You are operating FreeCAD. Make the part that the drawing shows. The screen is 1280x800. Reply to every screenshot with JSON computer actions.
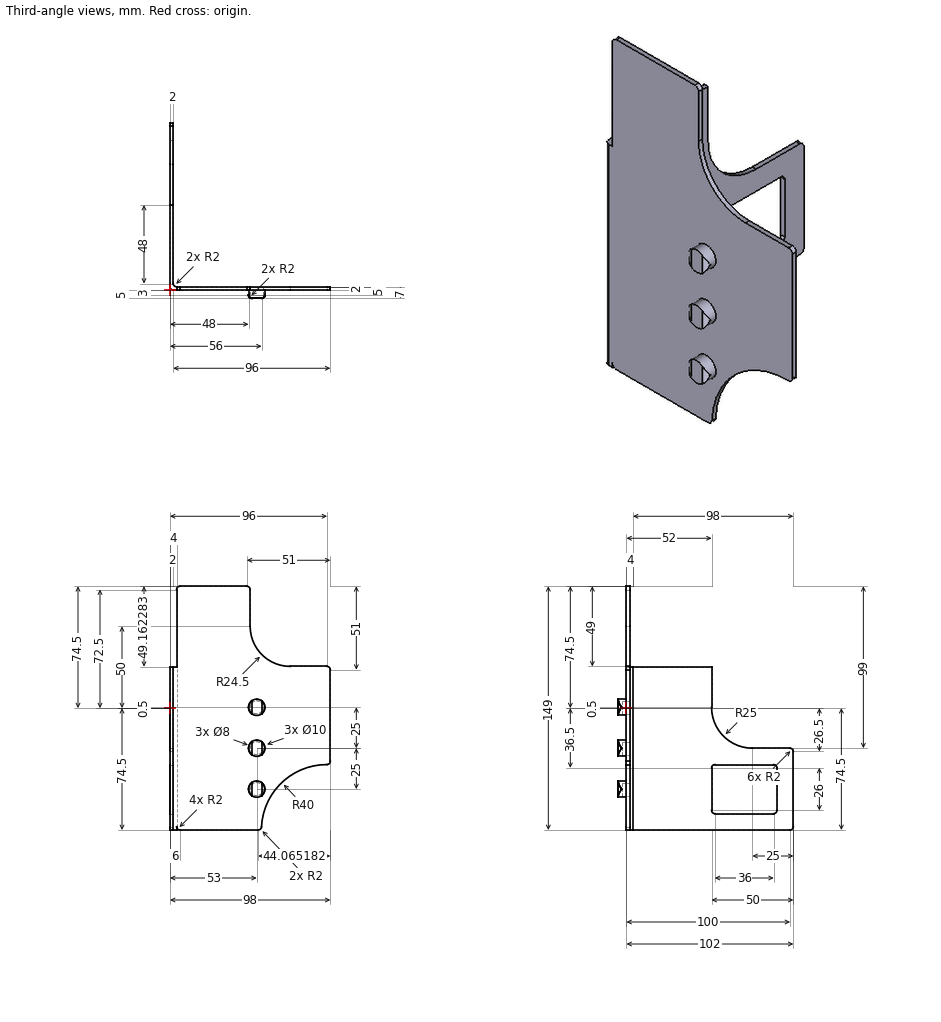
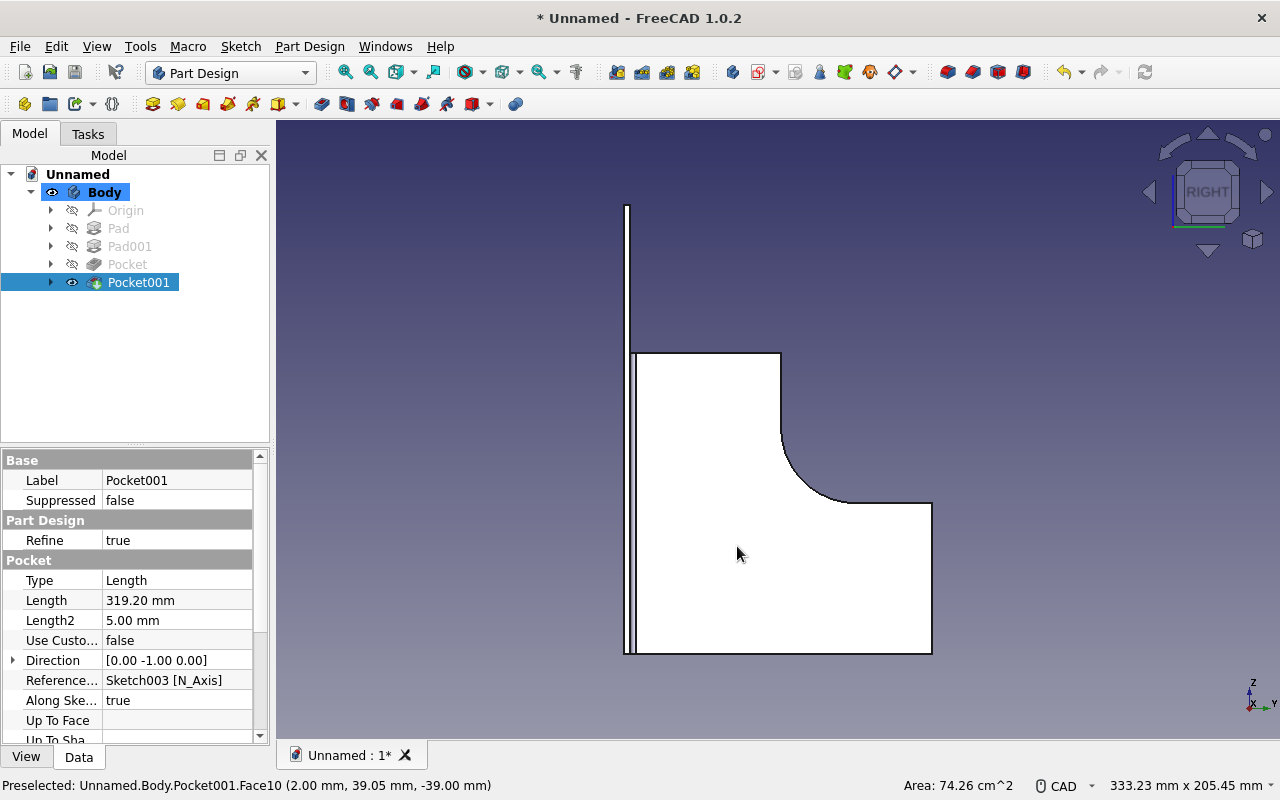
{"action": "left_click", "coordinate": [758, 72]}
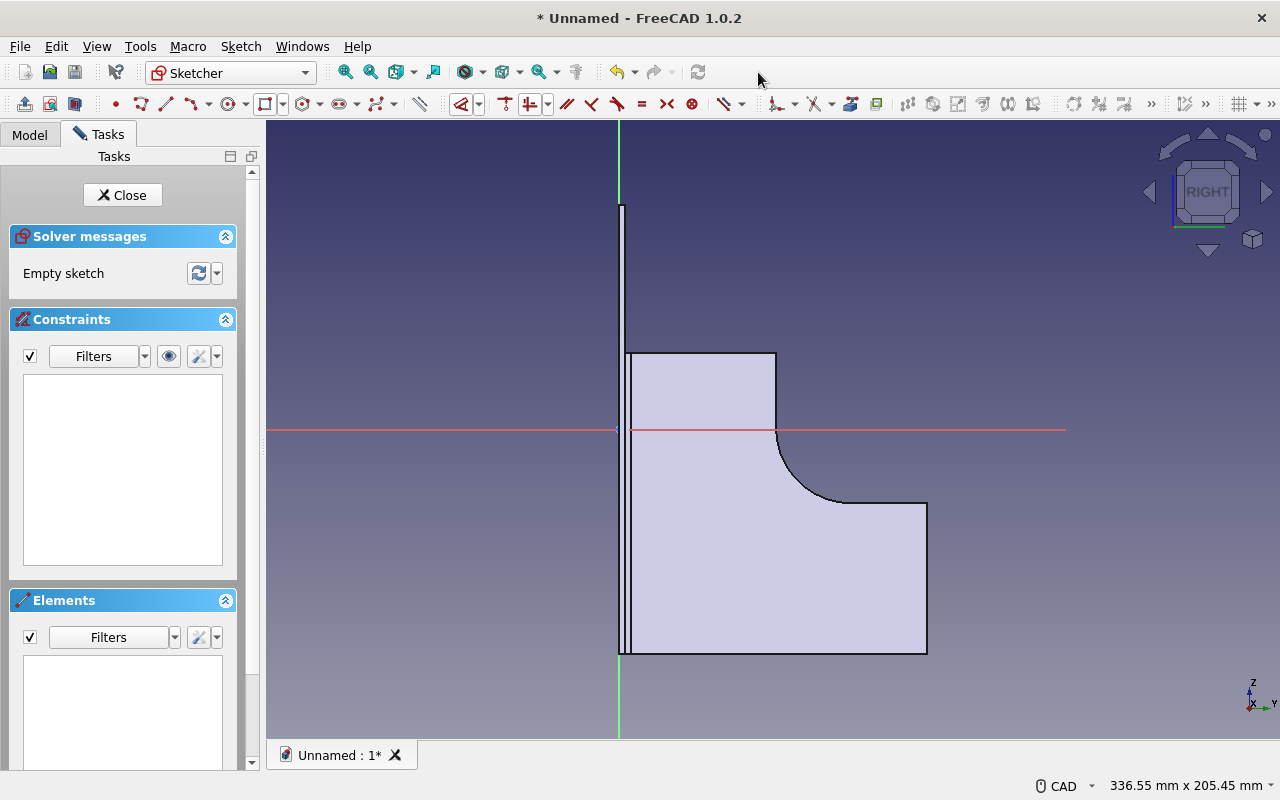
{"action": "key", "text": "q s"}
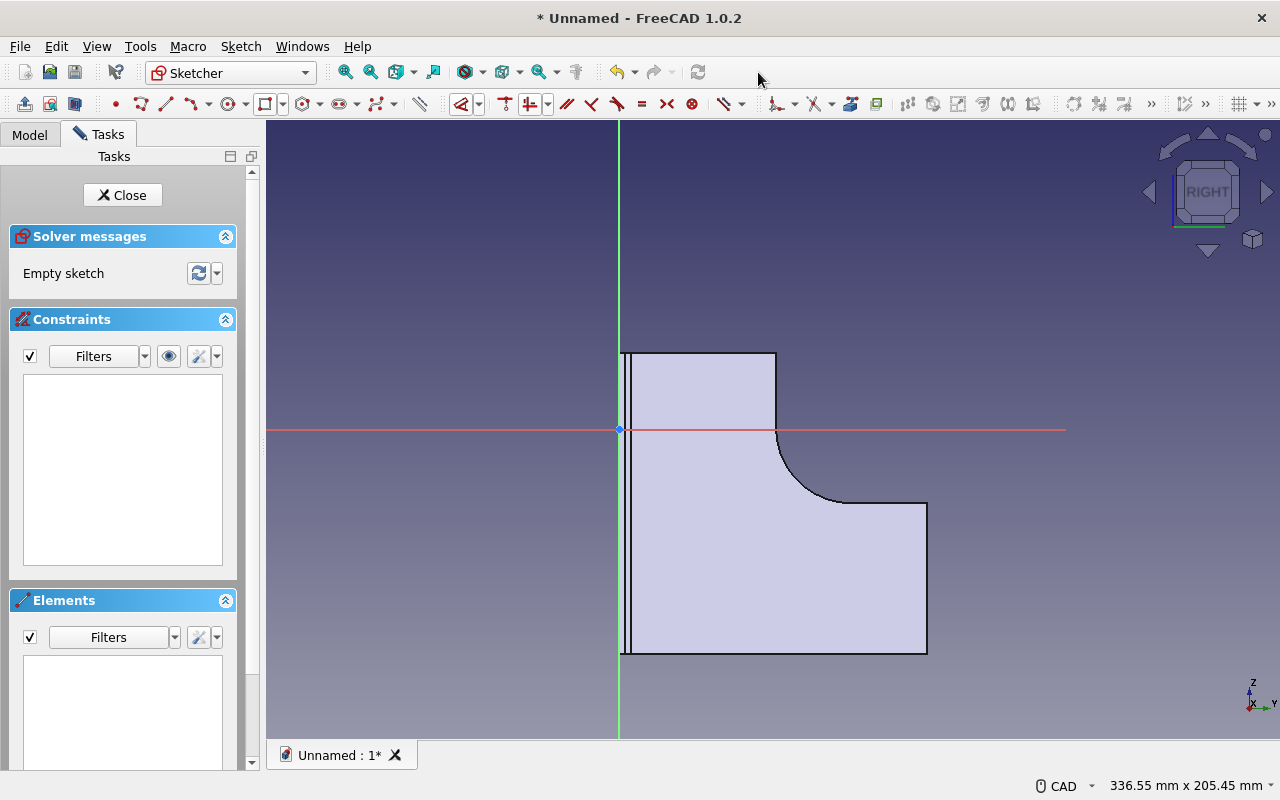
{"action": "scroll", "coordinate": [856, 678], "scroll_direction": "up", "scroll_amount": 3}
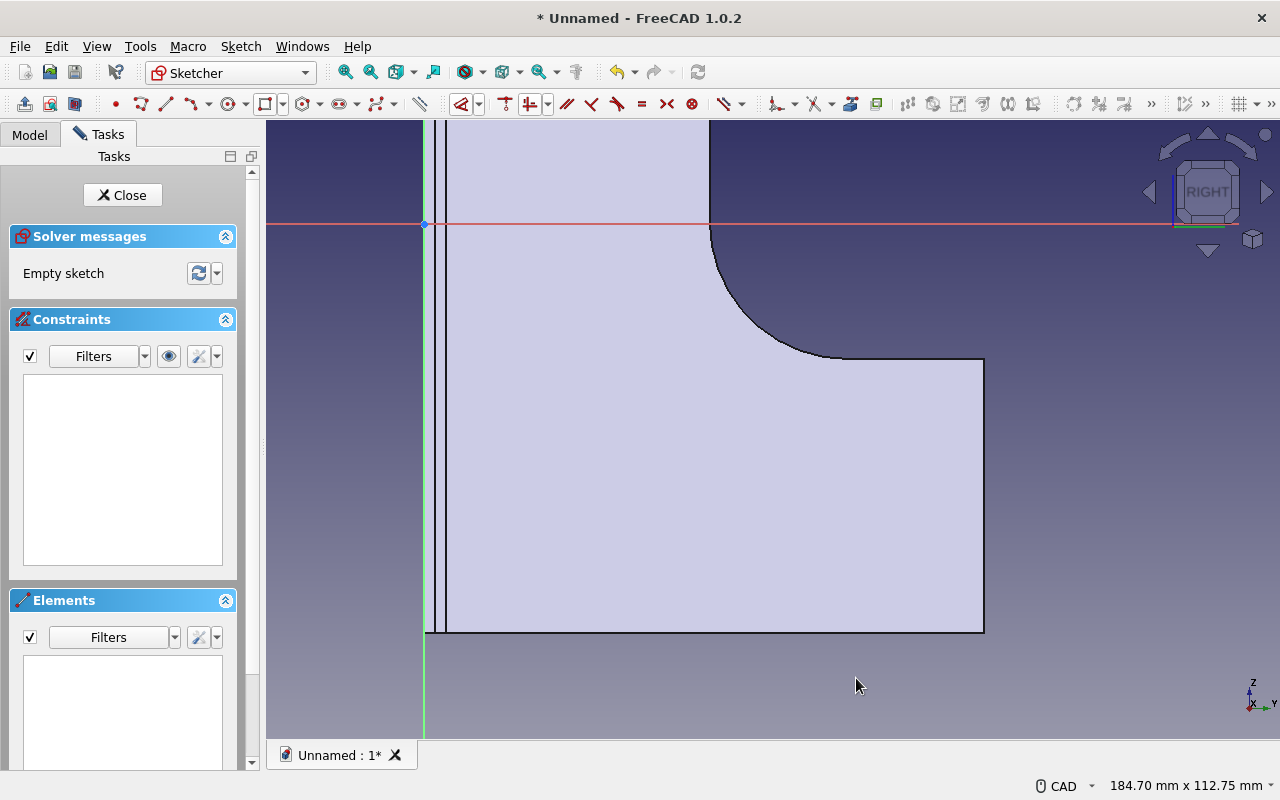
{"action": "left_click", "coordinate": [141, 104]}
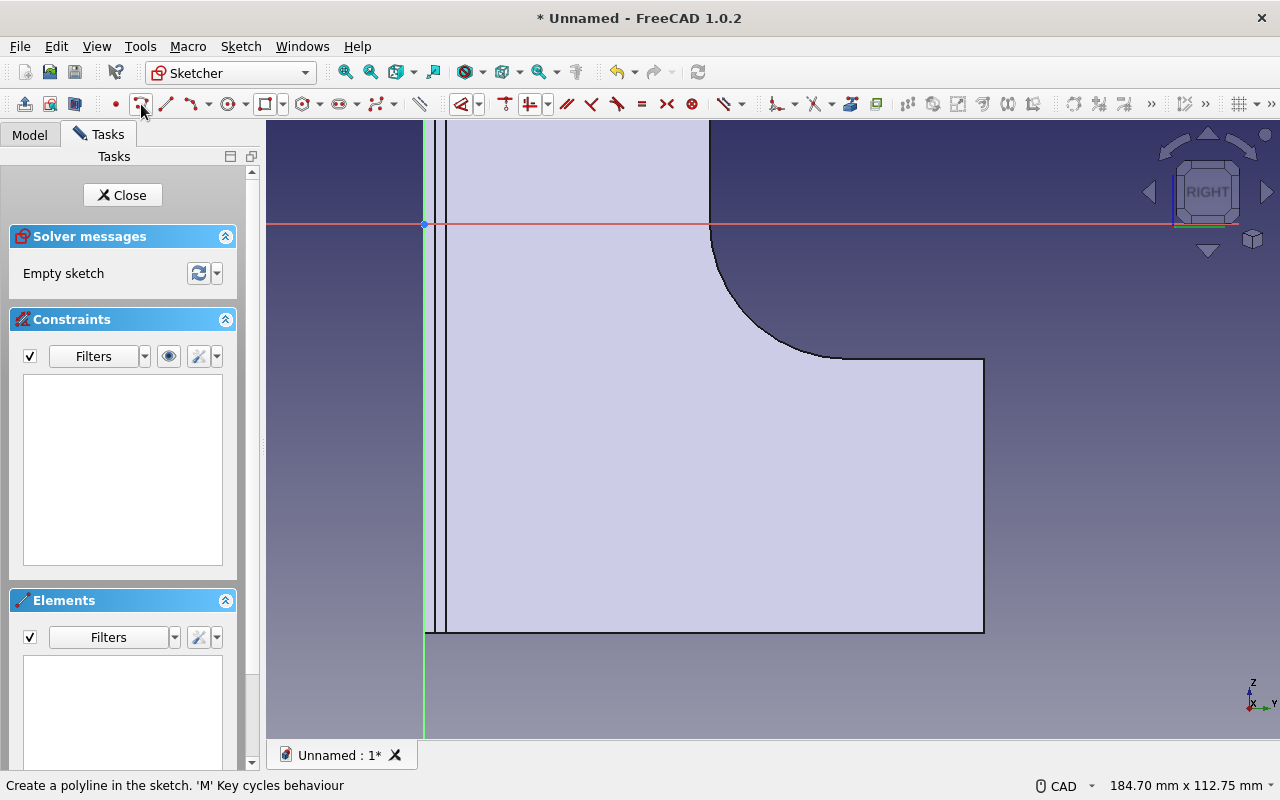
{"action": "left_click", "coordinate": [984, 370]}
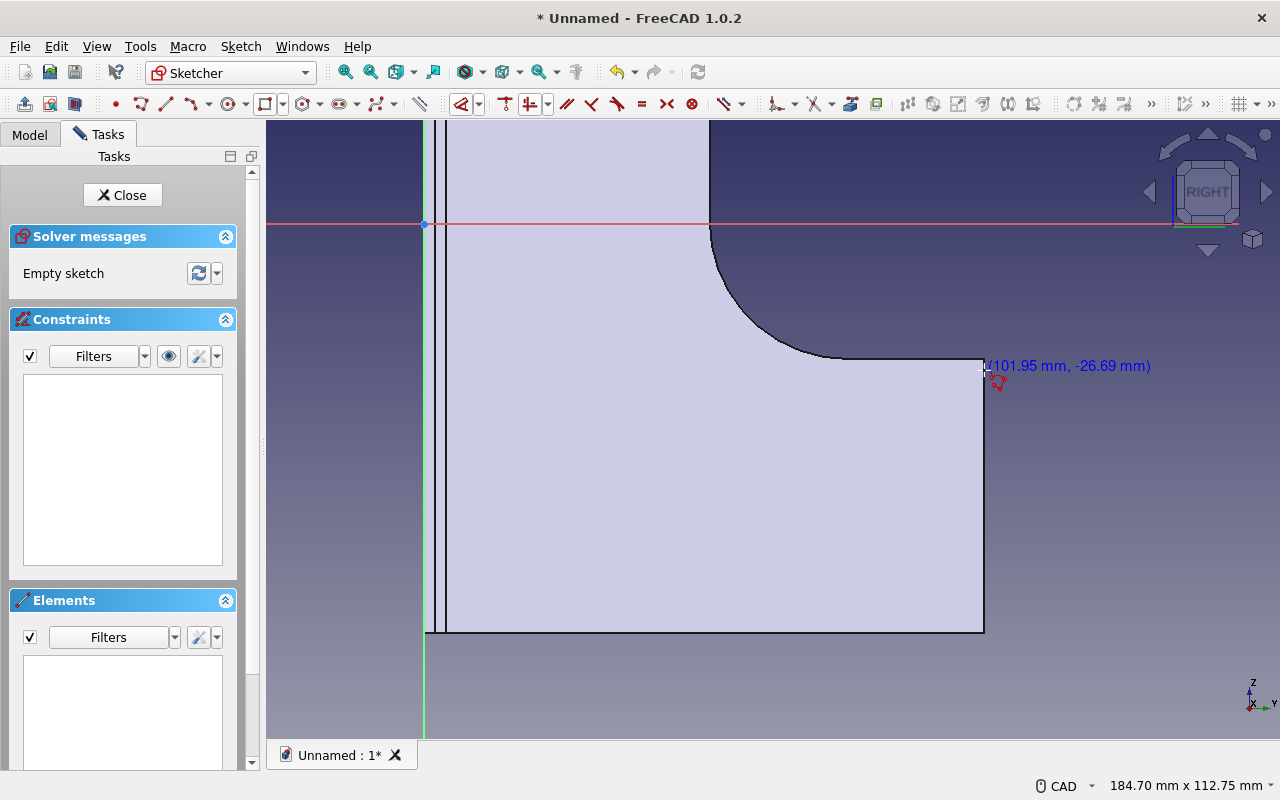
{"action": "scroll", "coordinate": [984, 359], "scroll_direction": "up", "scroll_amount": 2}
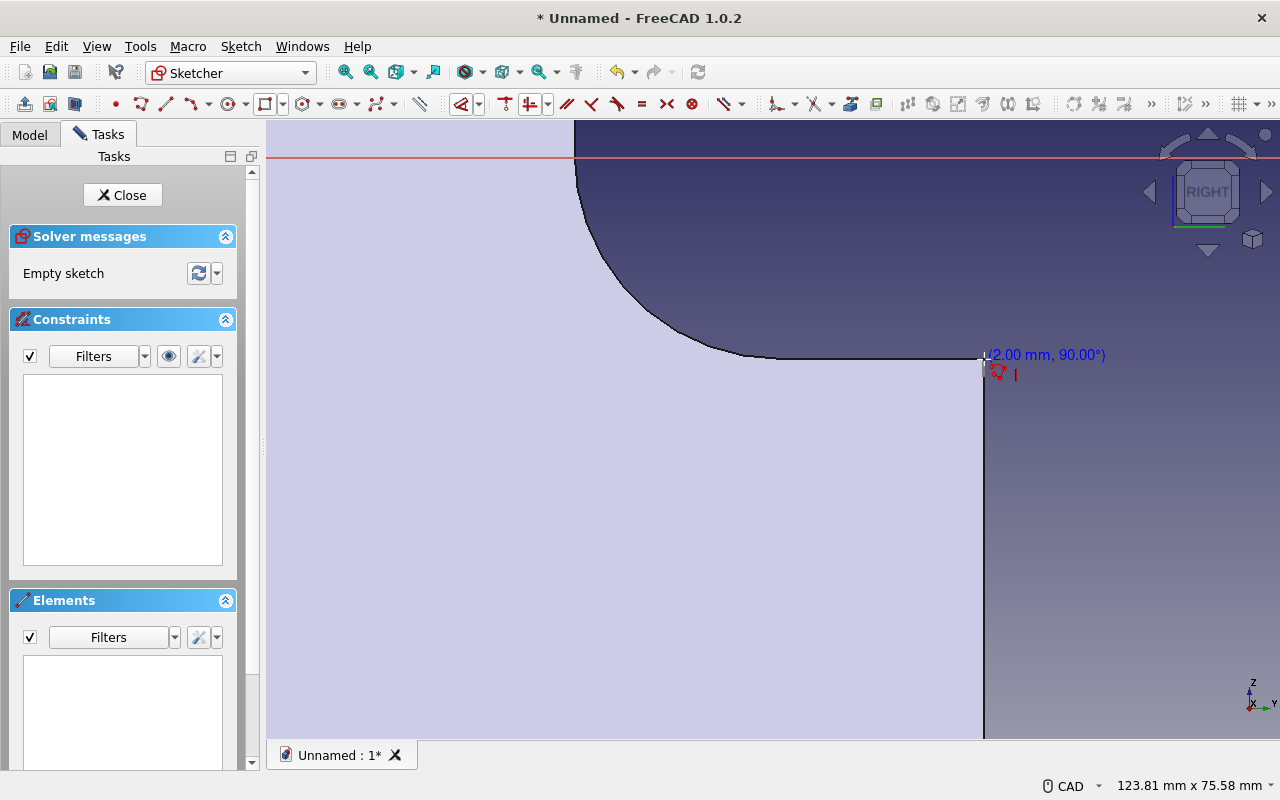
{"action": "left_click", "coordinate": [984, 359]}
{"action": "left_click", "coordinate": [968, 359]}
{"action": "right_click", "coordinate": [968, 359]}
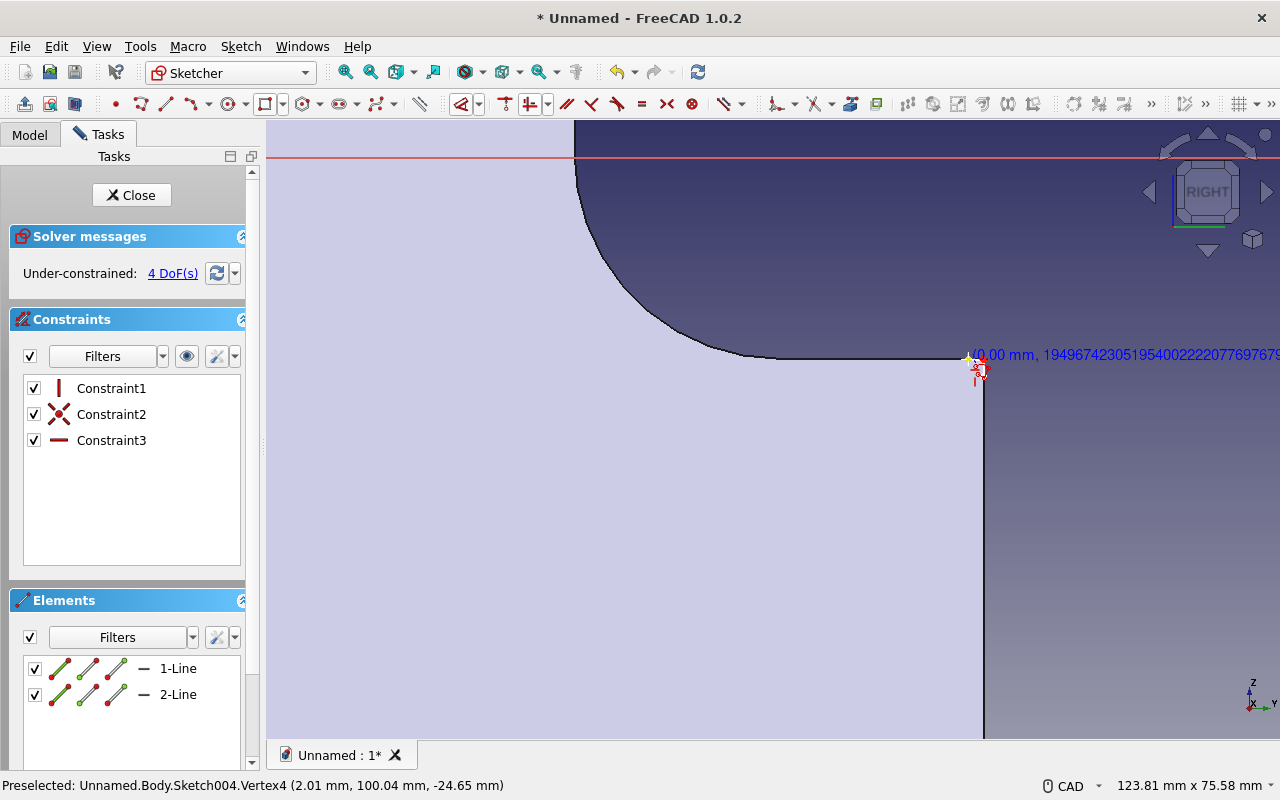
{"action": "left_click", "coordinate": [190, 104]}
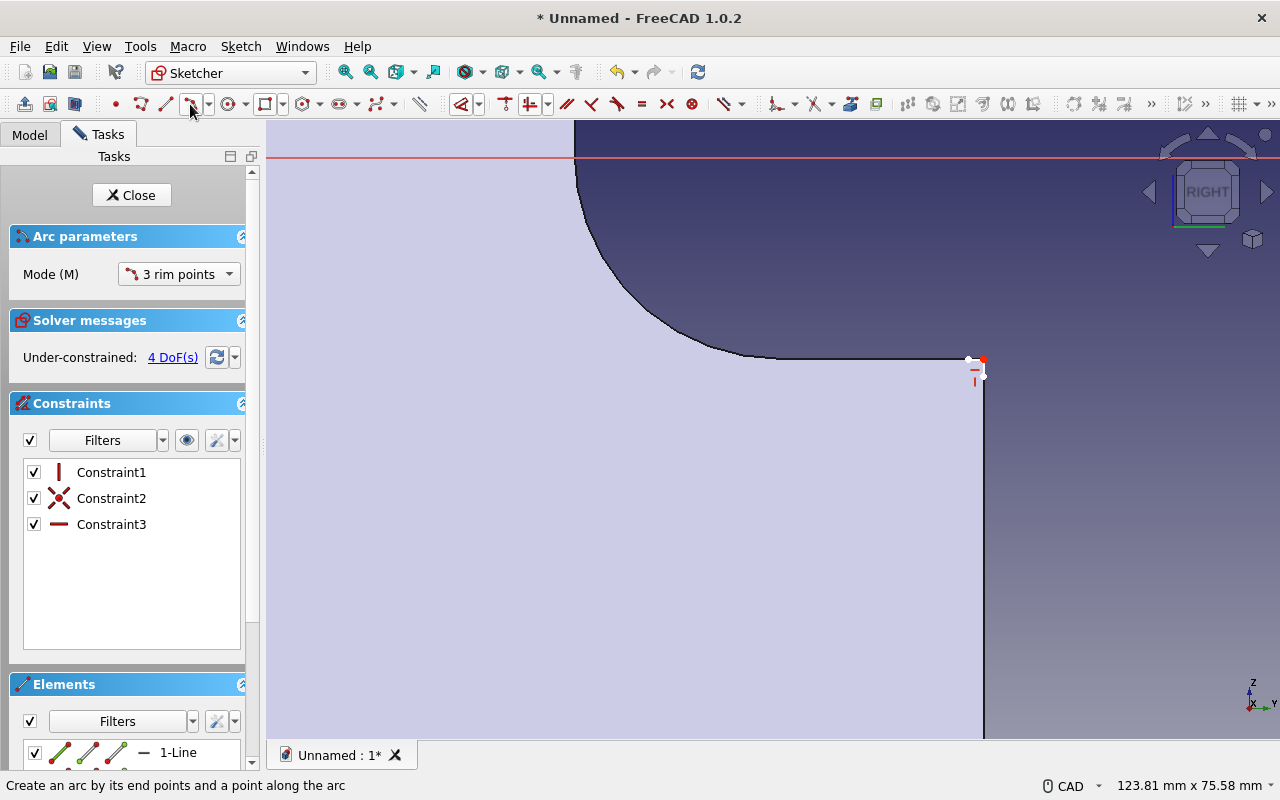
{"action": "scroll", "coordinate": [968, 359], "scroll_direction": "up", "scroll_amount": 4}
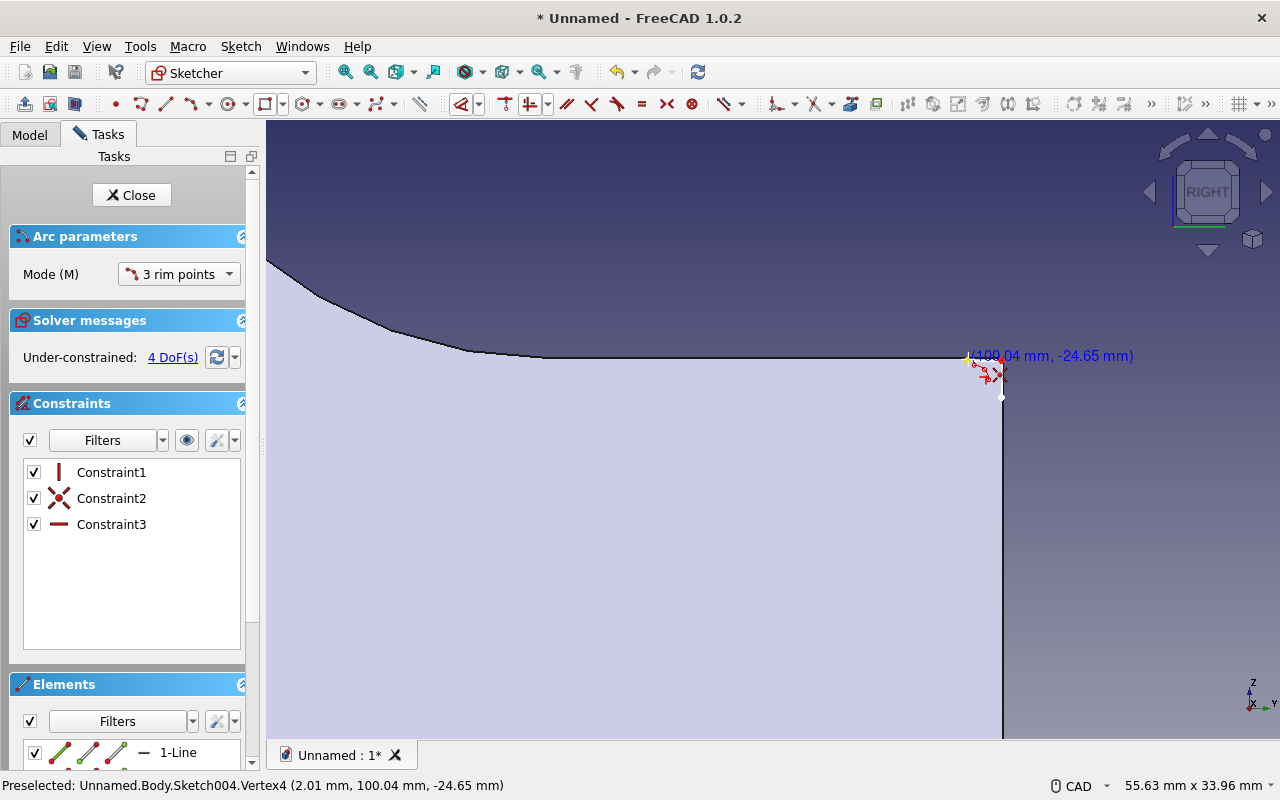
{"action": "left_click", "coordinate": [967, 361]}
{"action": "left_click", "coordinate": [1002, 398]}